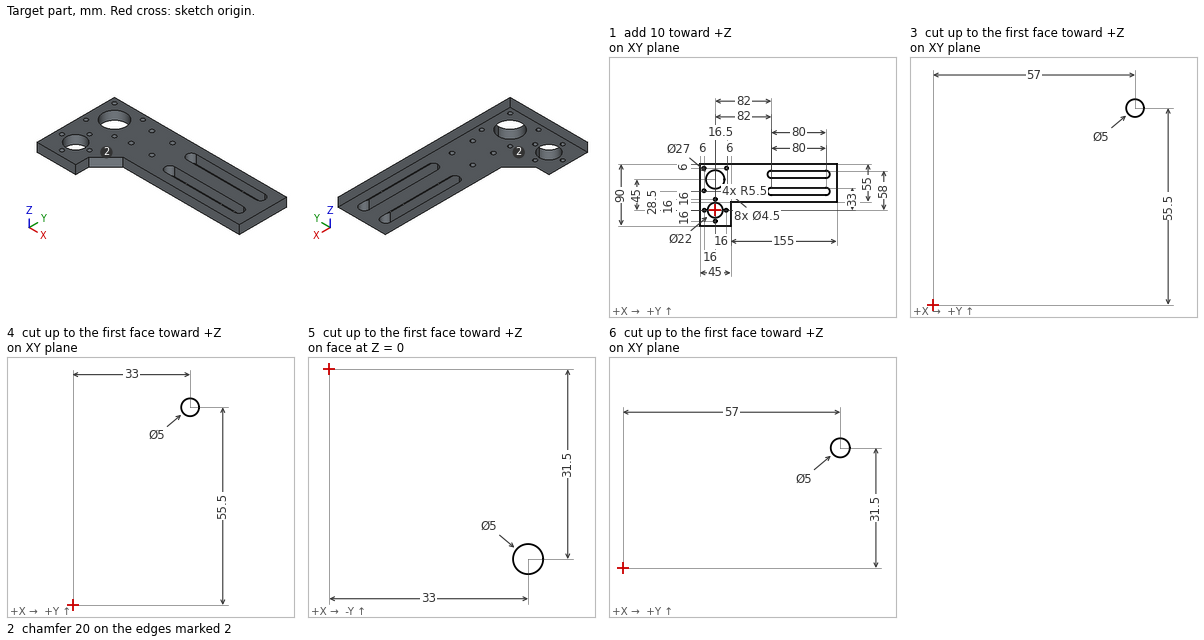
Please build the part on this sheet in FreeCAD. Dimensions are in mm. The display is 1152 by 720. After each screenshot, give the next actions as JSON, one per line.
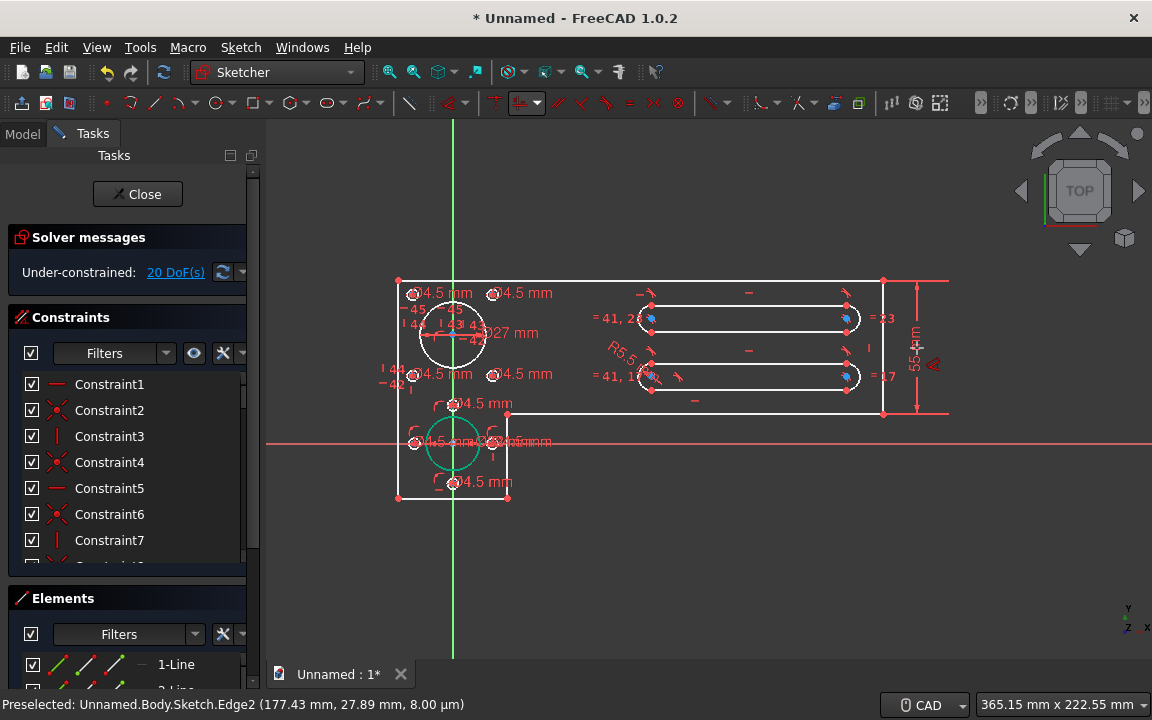
{"action": "left_click", "coordinate": [398, 346]}
{"action": "left_click", "coordinate": [364, 390]}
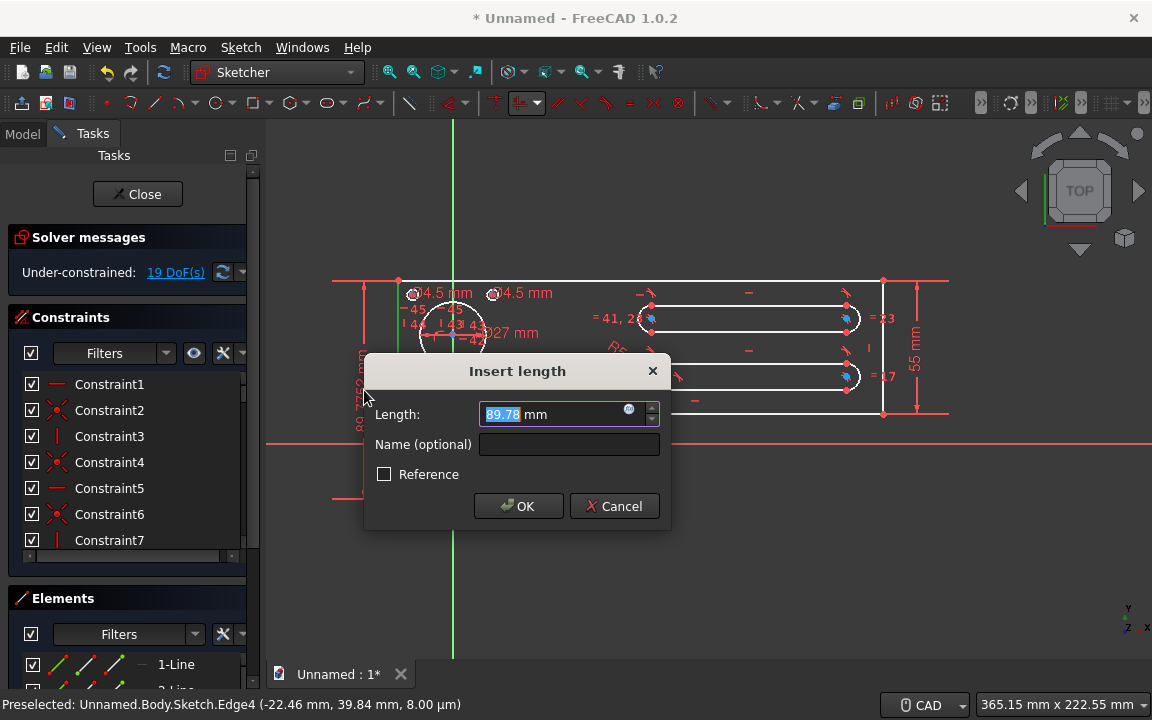
{"action": "type", "text": "90"}
{"action": "key", "text": "Return"}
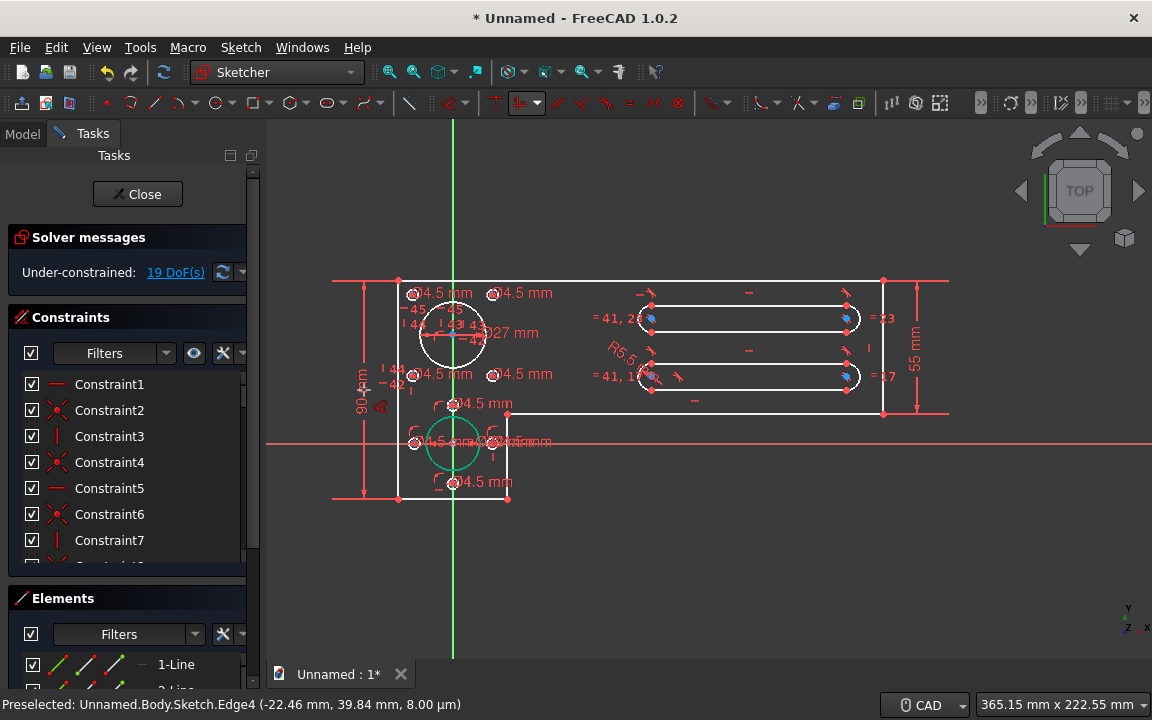
{"action": "left_click", "coordinate": [431, 499]}
{"action": "left_click", "coordinate": [428, 533]}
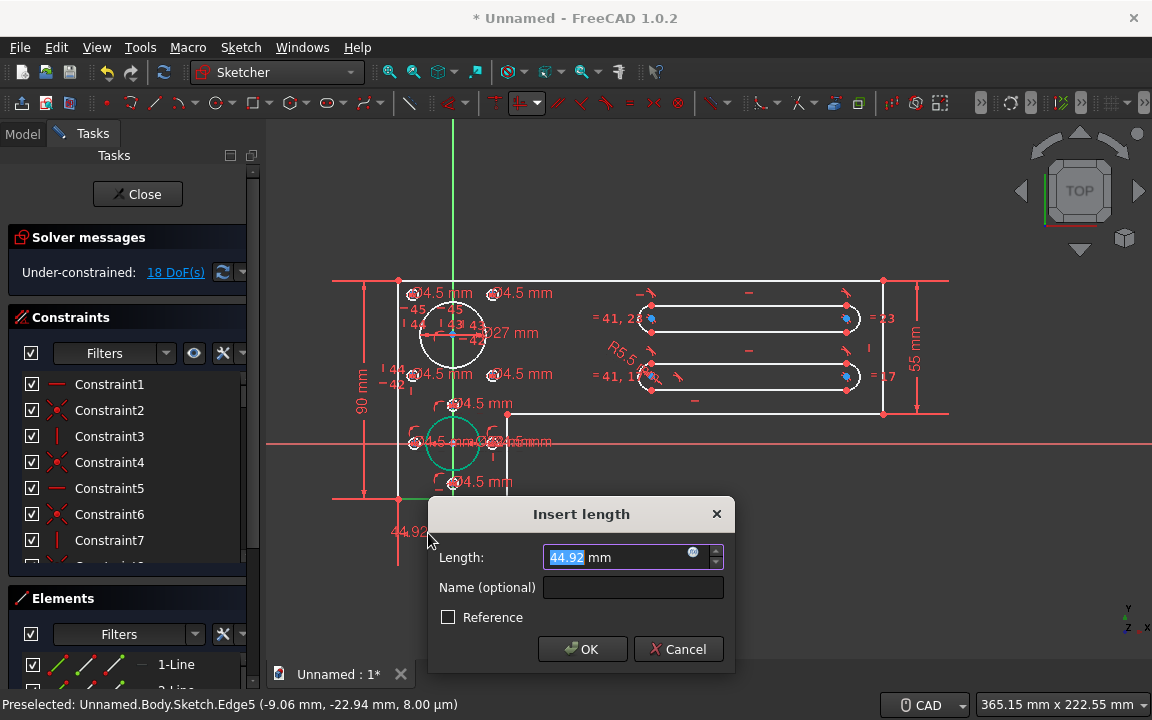
{"action": "type", "text": "45"}
{"action": "key", "text": "Return"}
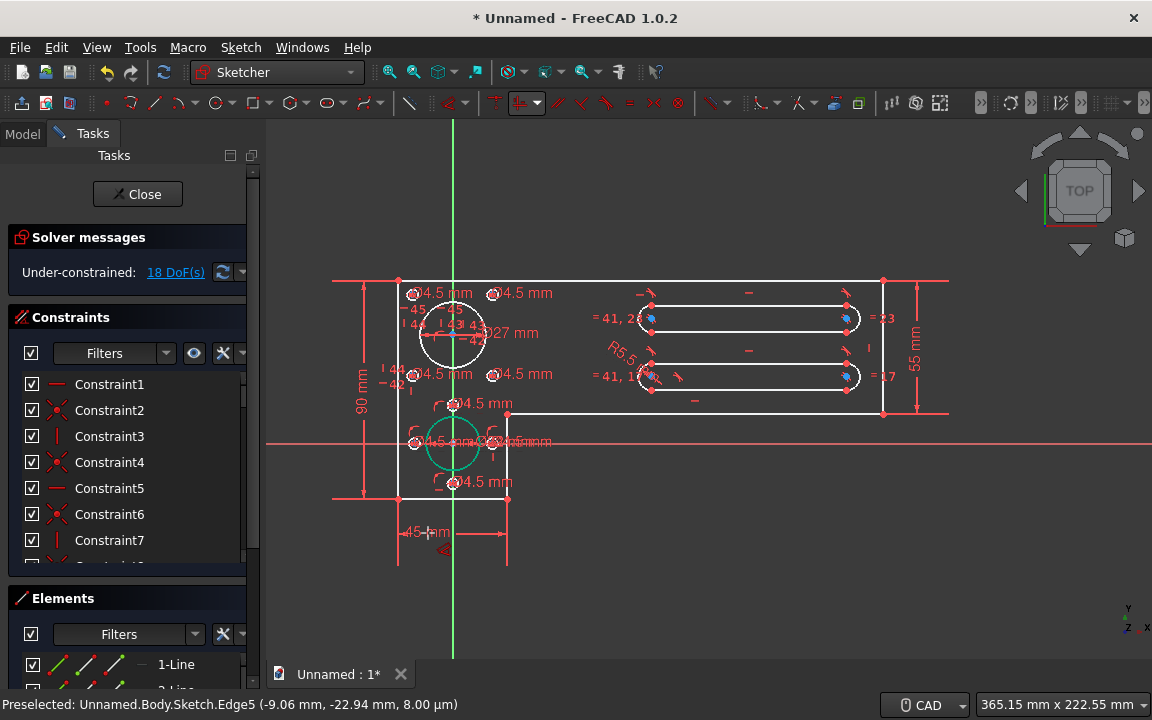
{"action": "left_click", "coordinate": [710, 364]}
{"action": "left_click", "coordinate": [749, 258]}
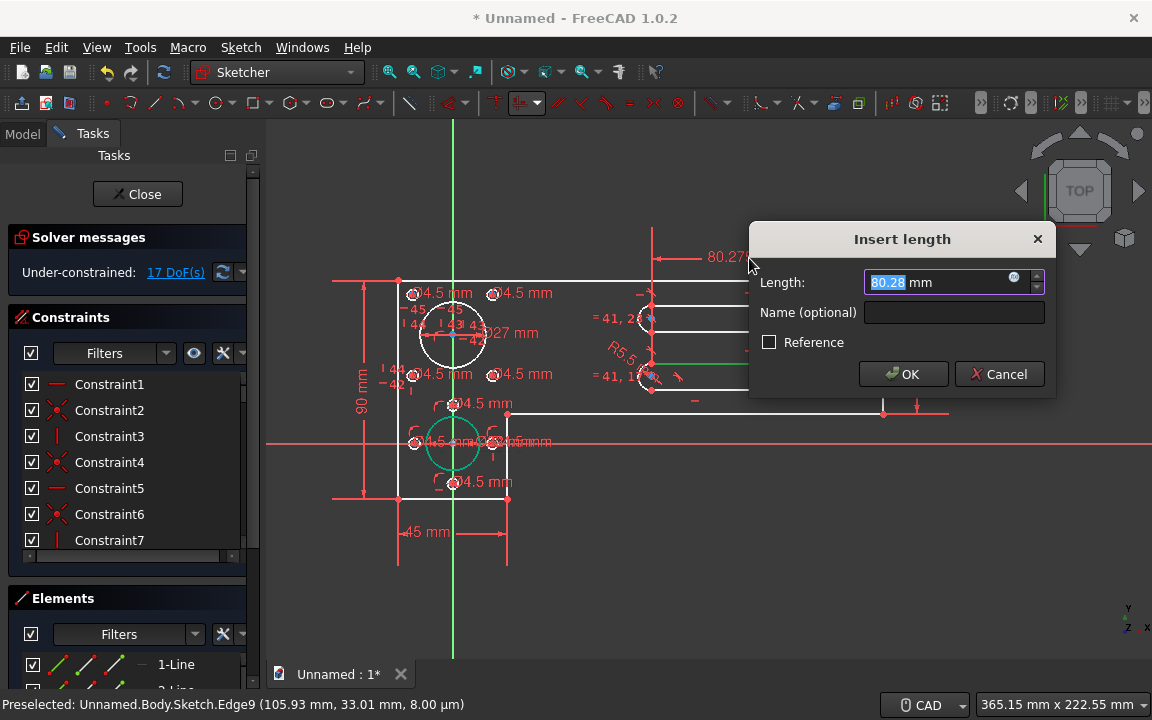
{"action": "type", "text": "80"}
{"action": "key", "text": "Return"}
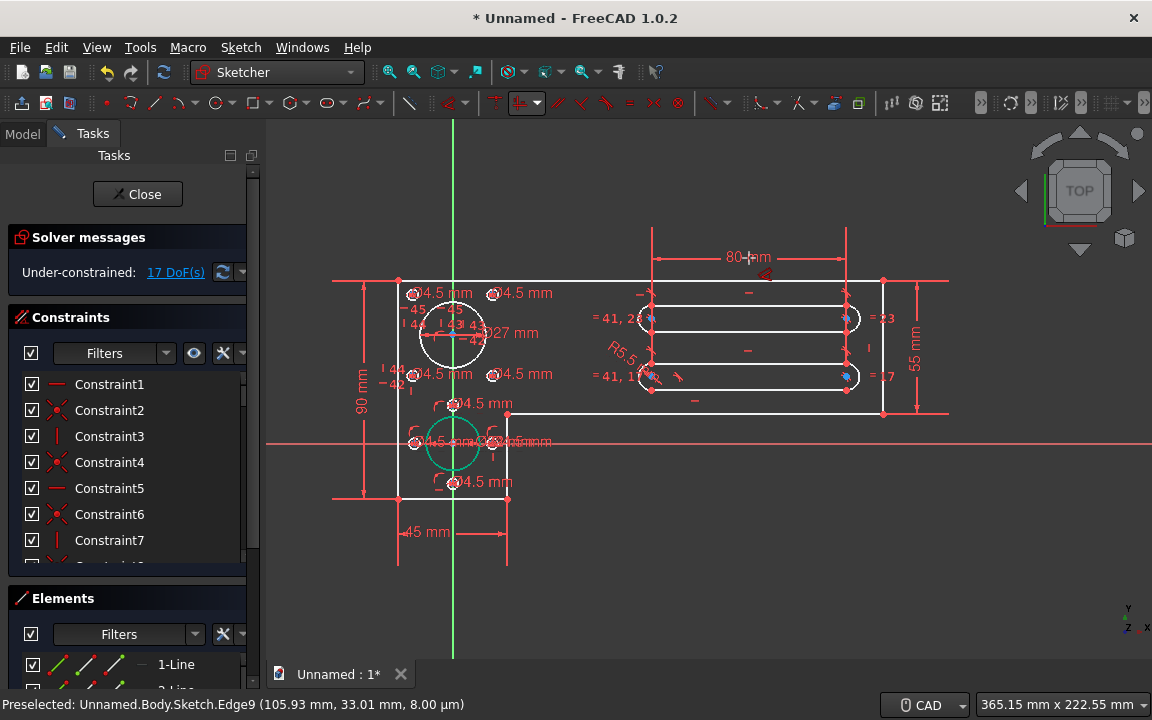
{"action": "left_click", "coordinate": [710, 306]}
{"action": "left_click", "coordinate": [749, 224]}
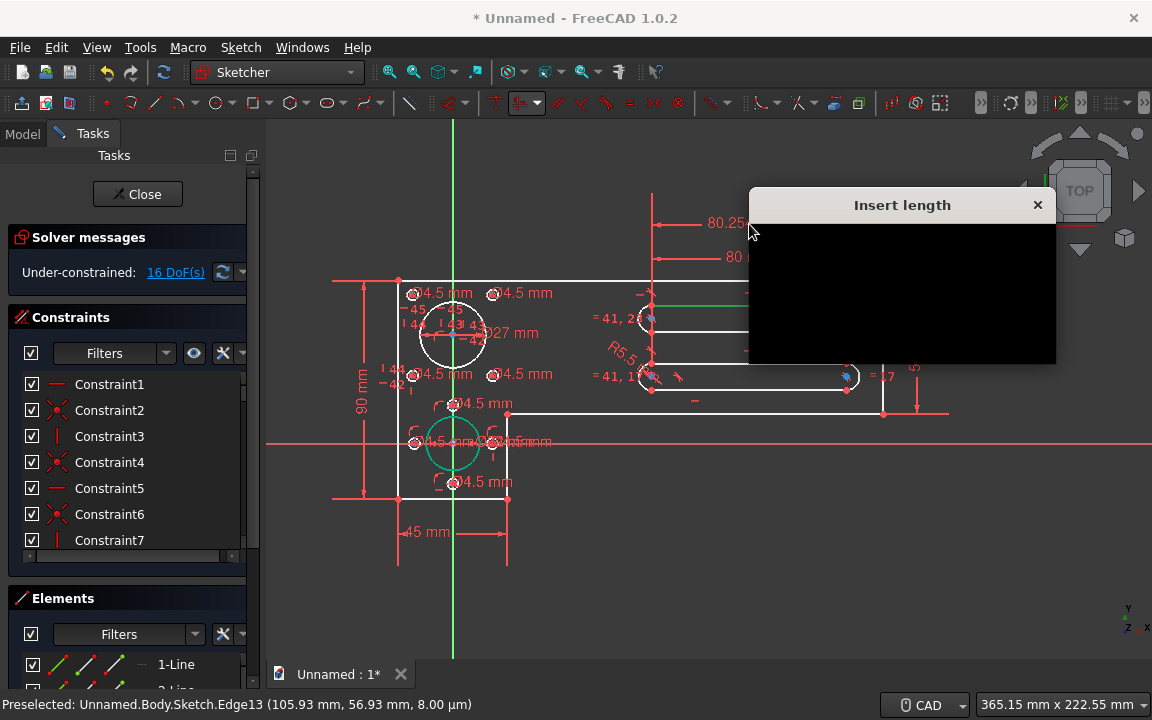
{"action": "type", "text": "80"}
{"action": "key", "text": "Return"}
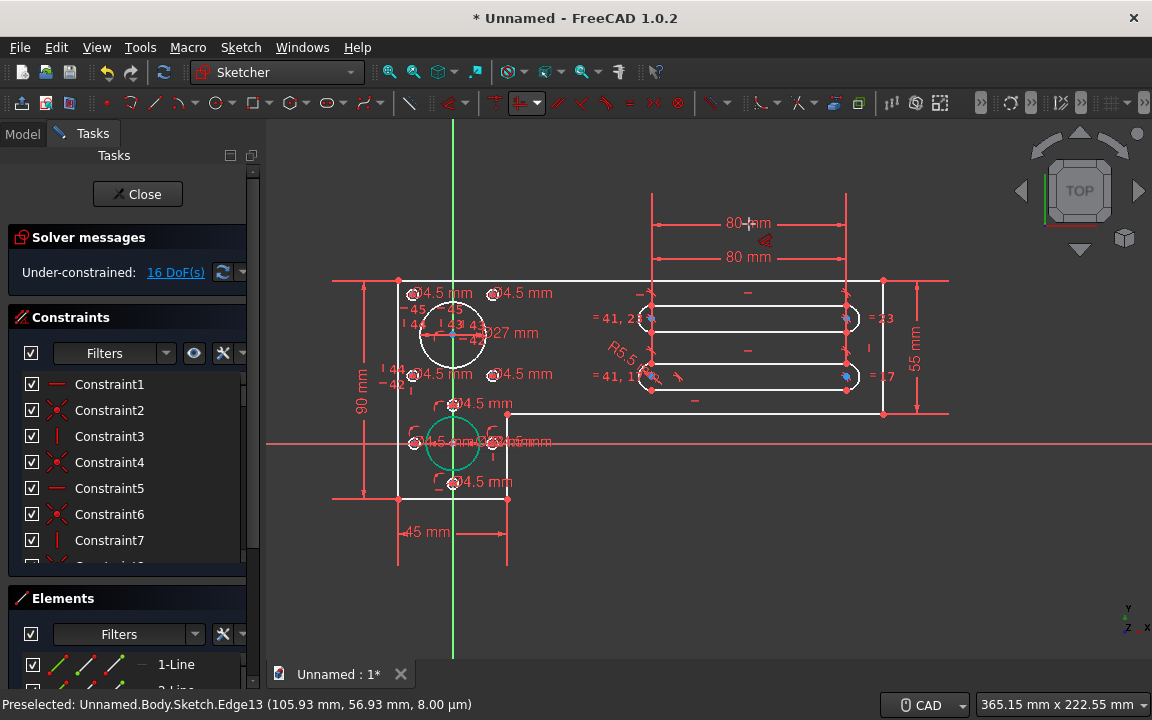
{"action": "left_click", "coordinate": [453, 484]}
{"action": "left_click", "coordinate": [419, 473]}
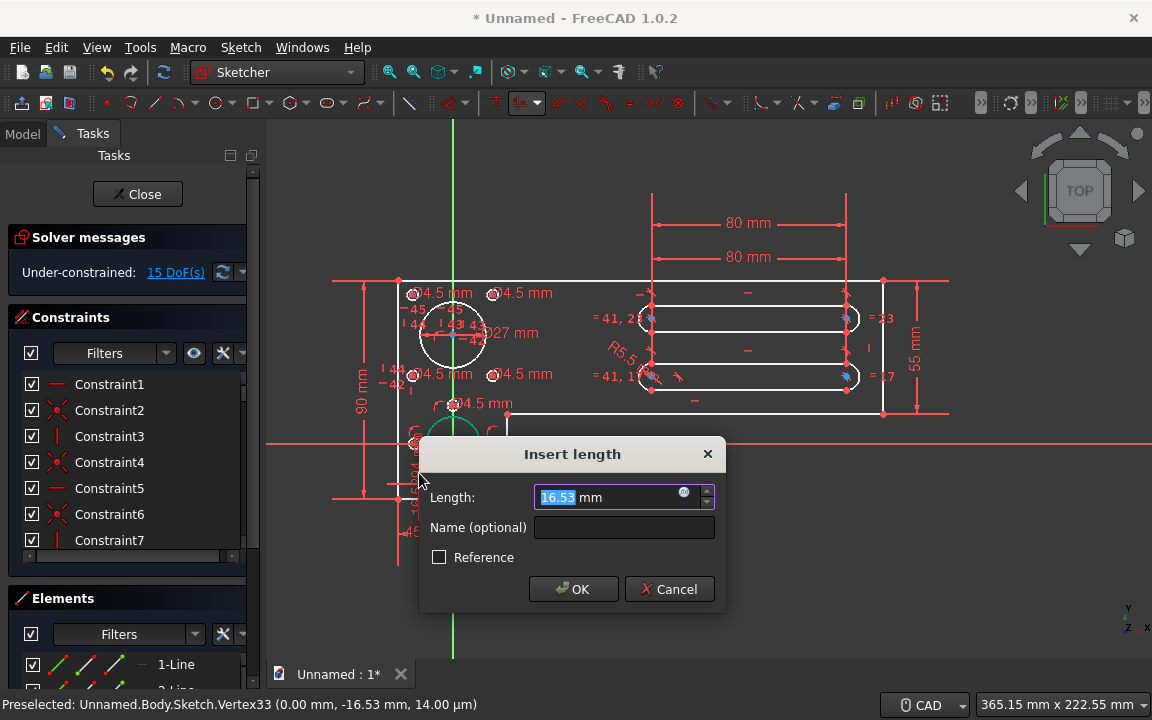
{"action": "type", "text": "16"}
{"action": "key", "text": "Return"}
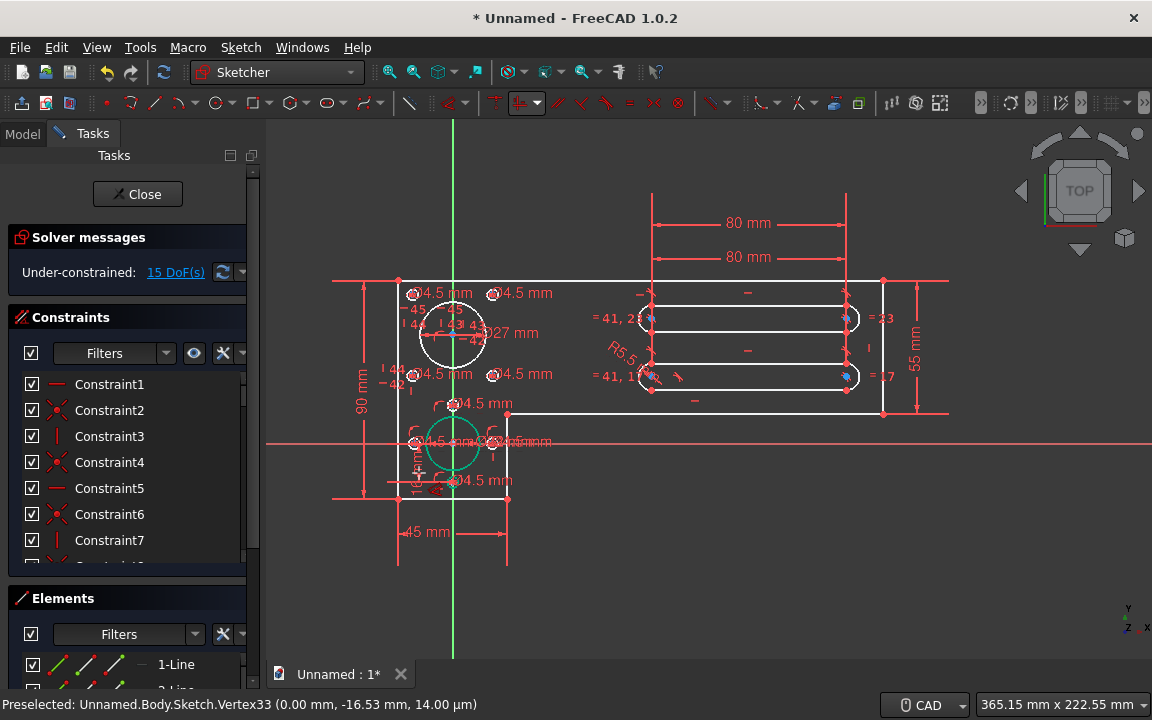
{"action": "left_click", "coordinate": [492, 444]}
{"action": "left_click", "coordinate": [482, 410]}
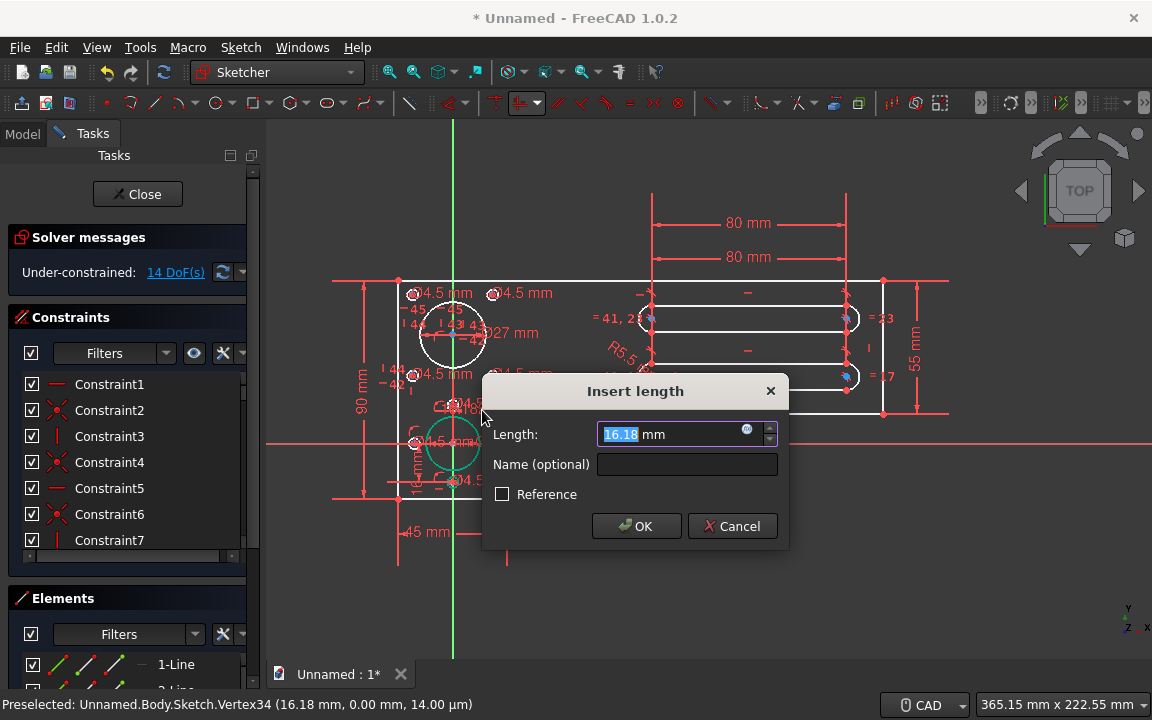
{"action": "type", "text": "16"}
{"action": "key", "text": "Return"}